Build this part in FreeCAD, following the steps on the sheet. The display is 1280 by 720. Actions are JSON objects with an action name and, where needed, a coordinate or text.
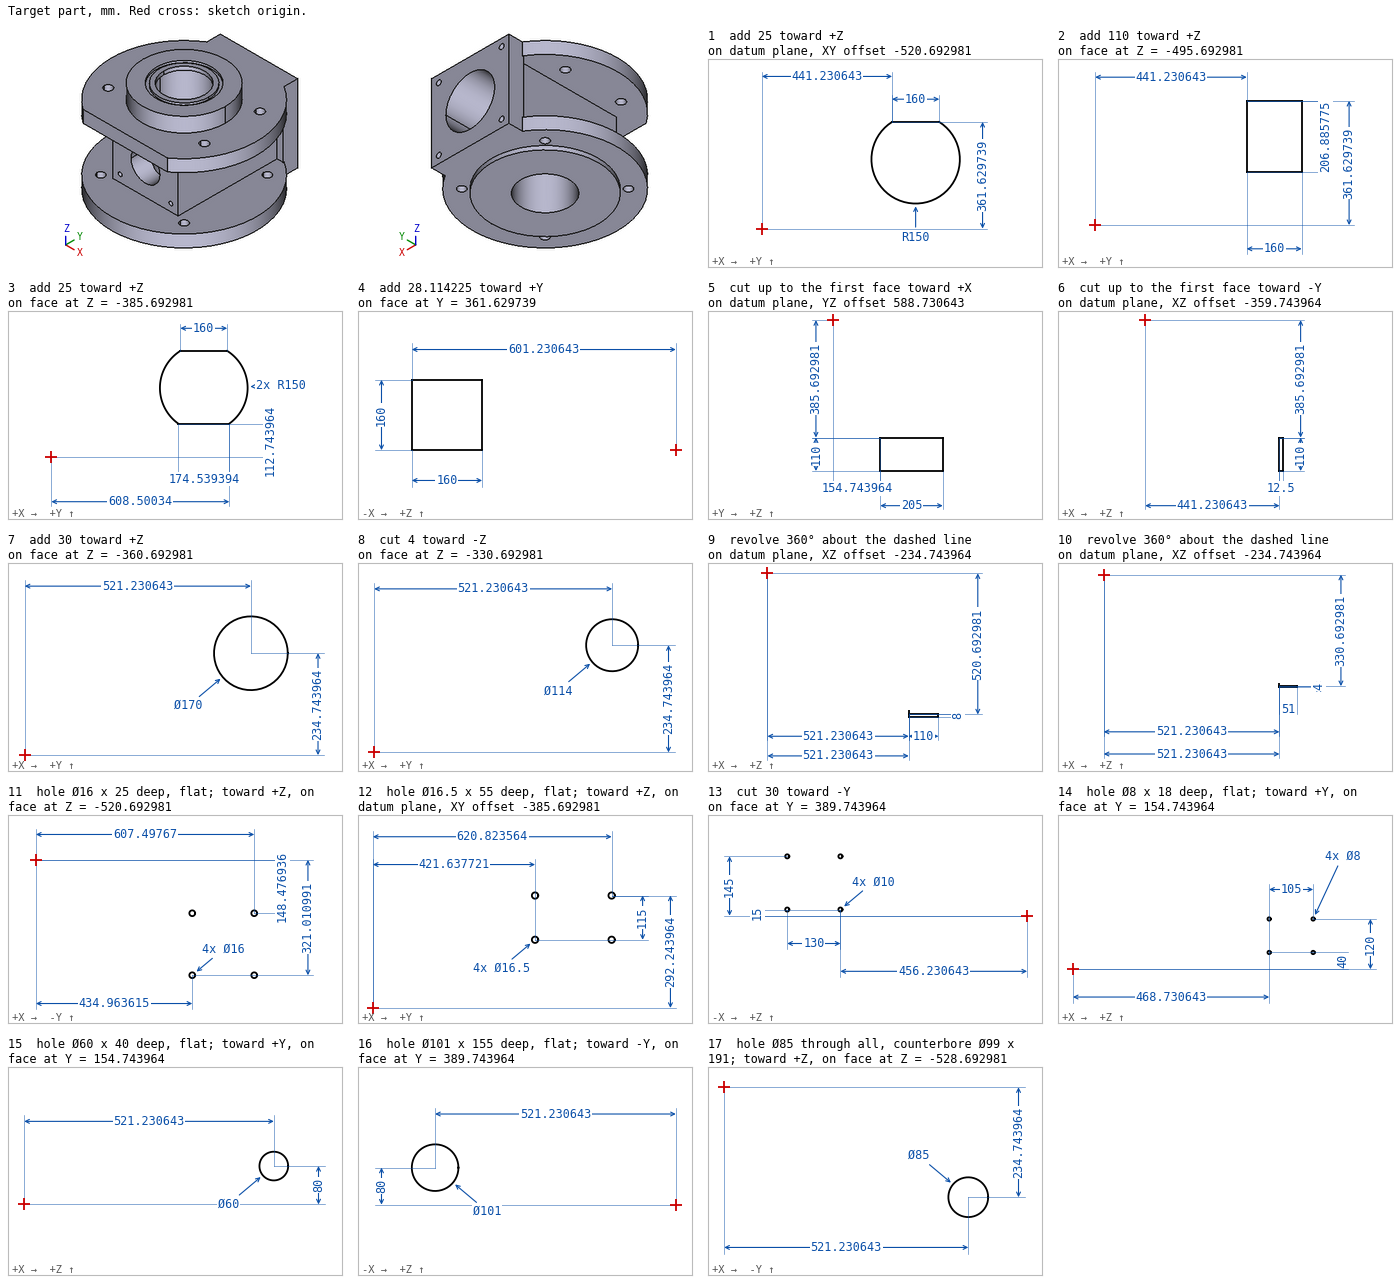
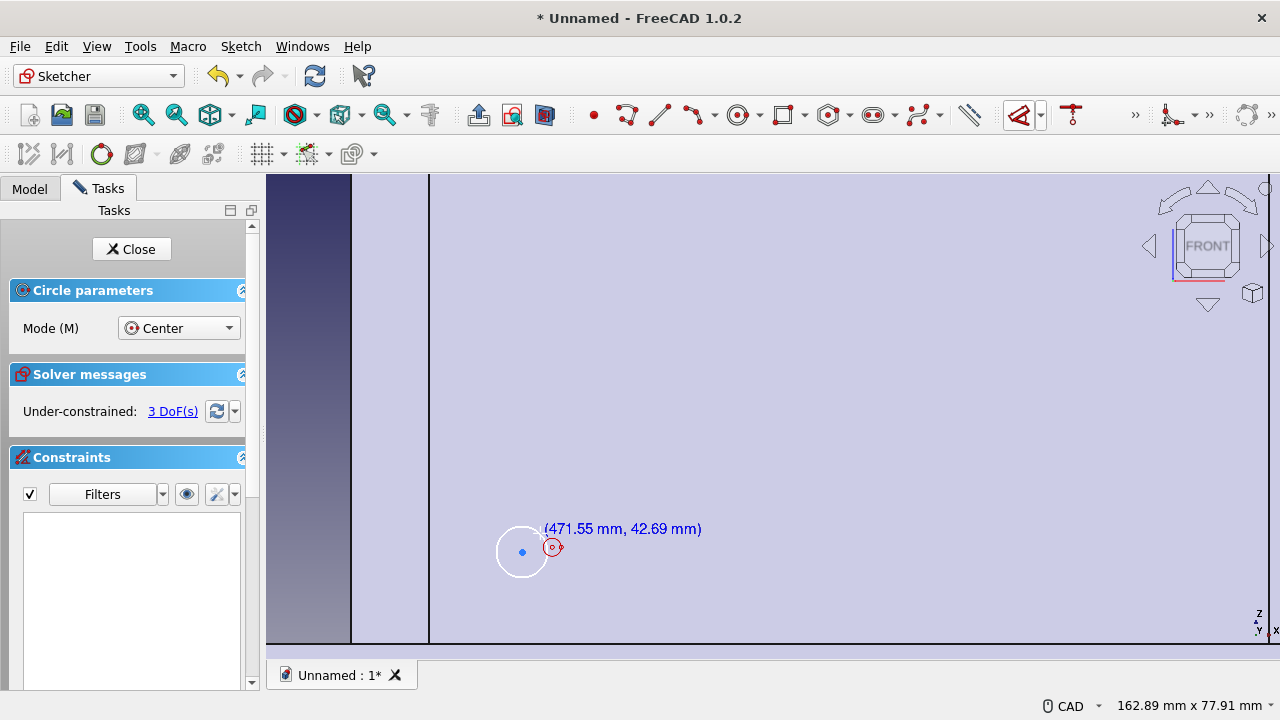
{"action": "scroll", "coordinate": [528, 556], "scroll_direction": "down", "scroll_amount": 3}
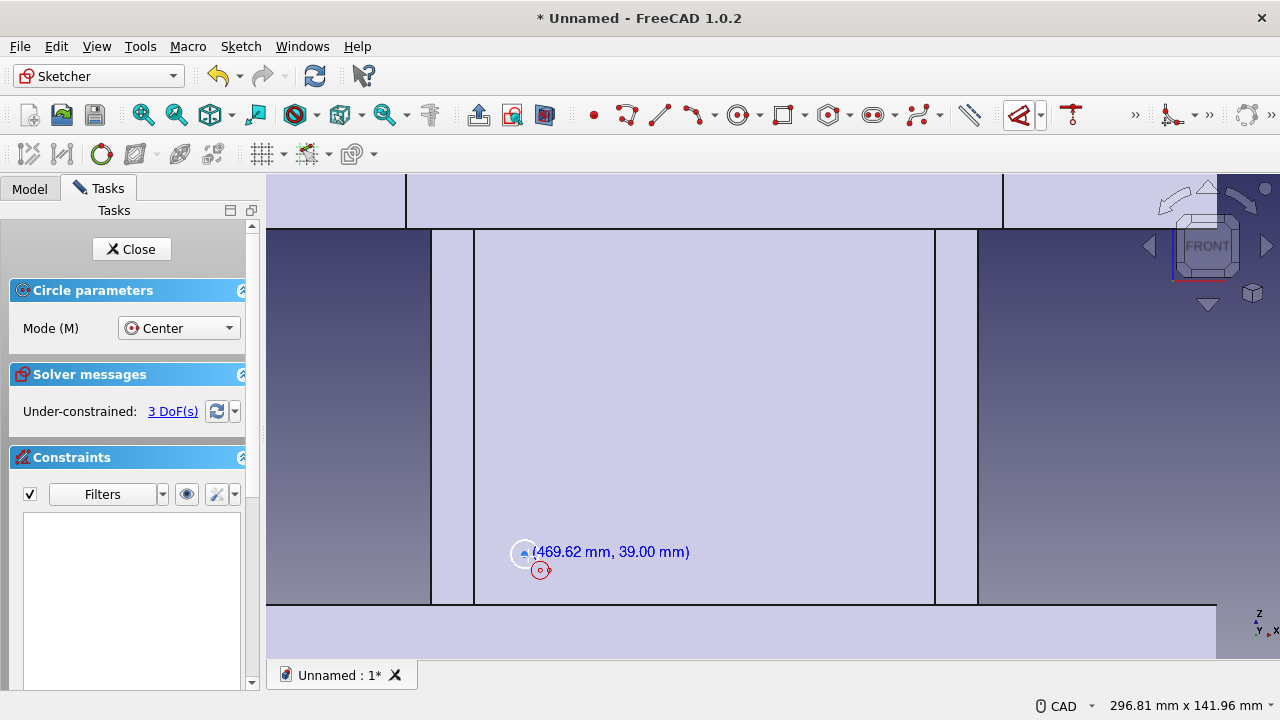
{"action": "scroll", "coordinate": [884, 280], "scroll_direction": "up", "scroll_amount": 3}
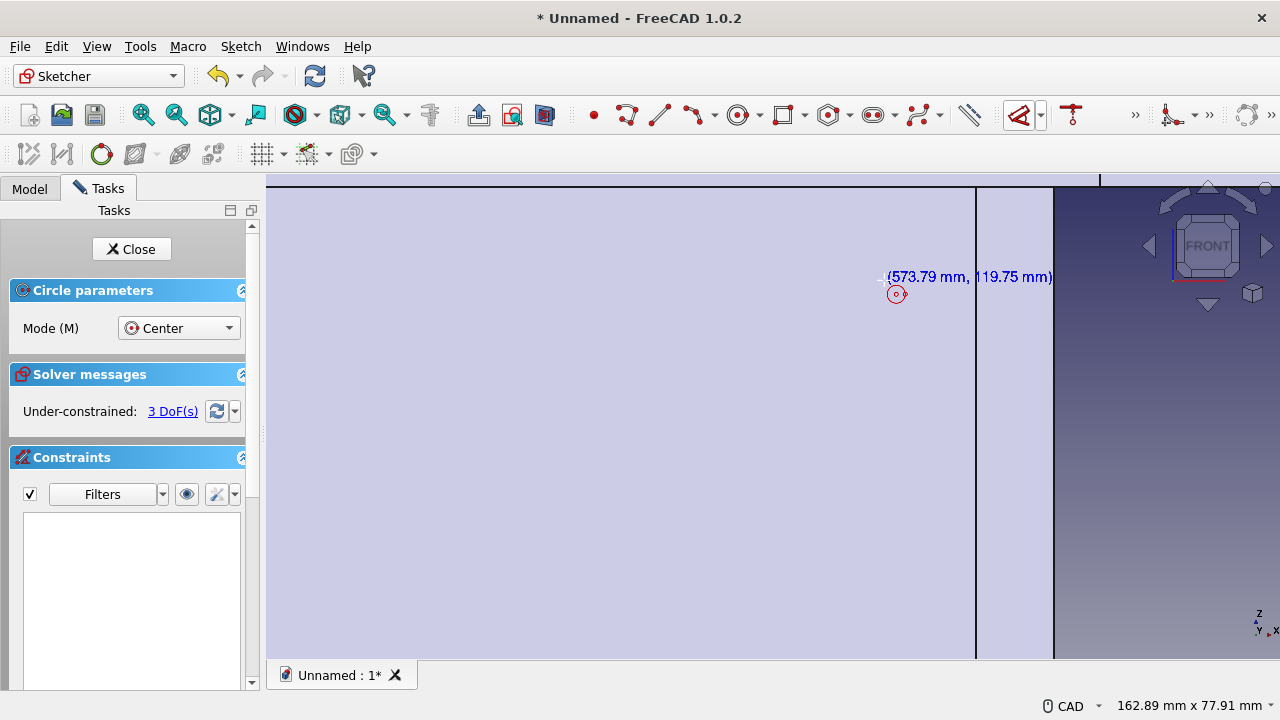
{"action": "left_click", "coordinate": [883, 280]}
{"action": "left_click", "coordinate": [901, 263]}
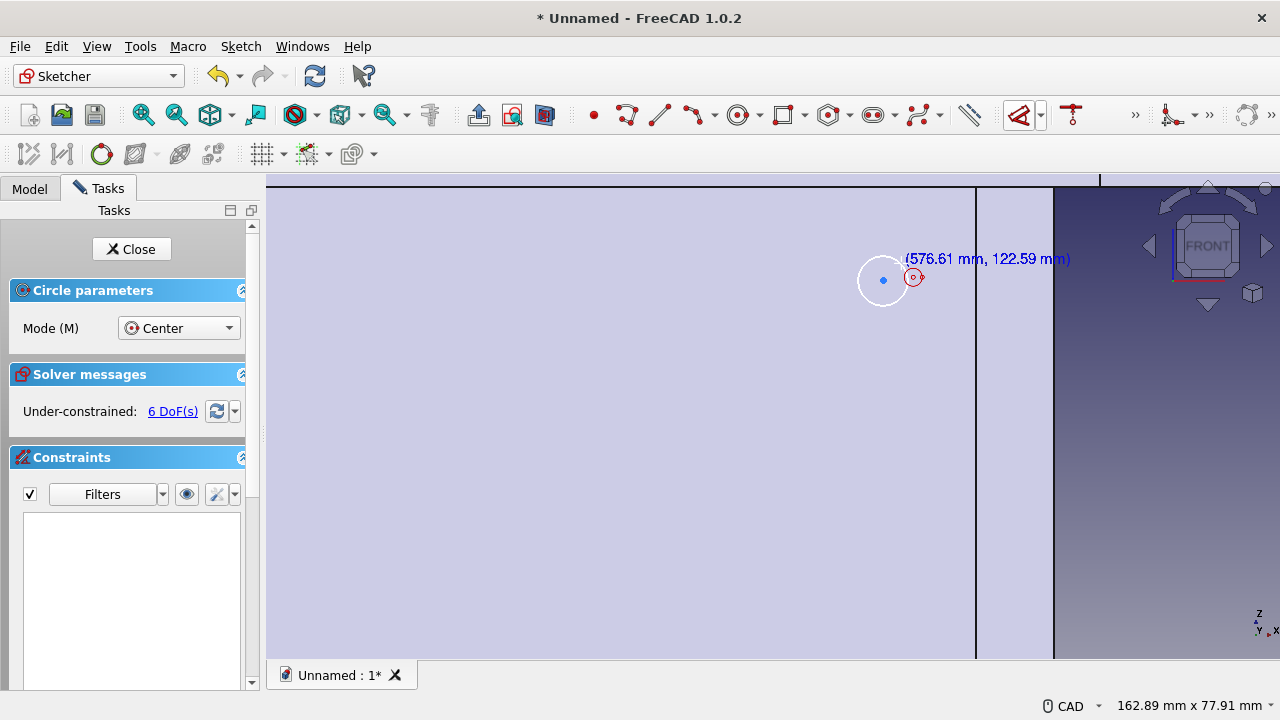
{"action": "scroll", "coordinate": [885, 280], "scroll_direction": "down", "scroll_amount": 3}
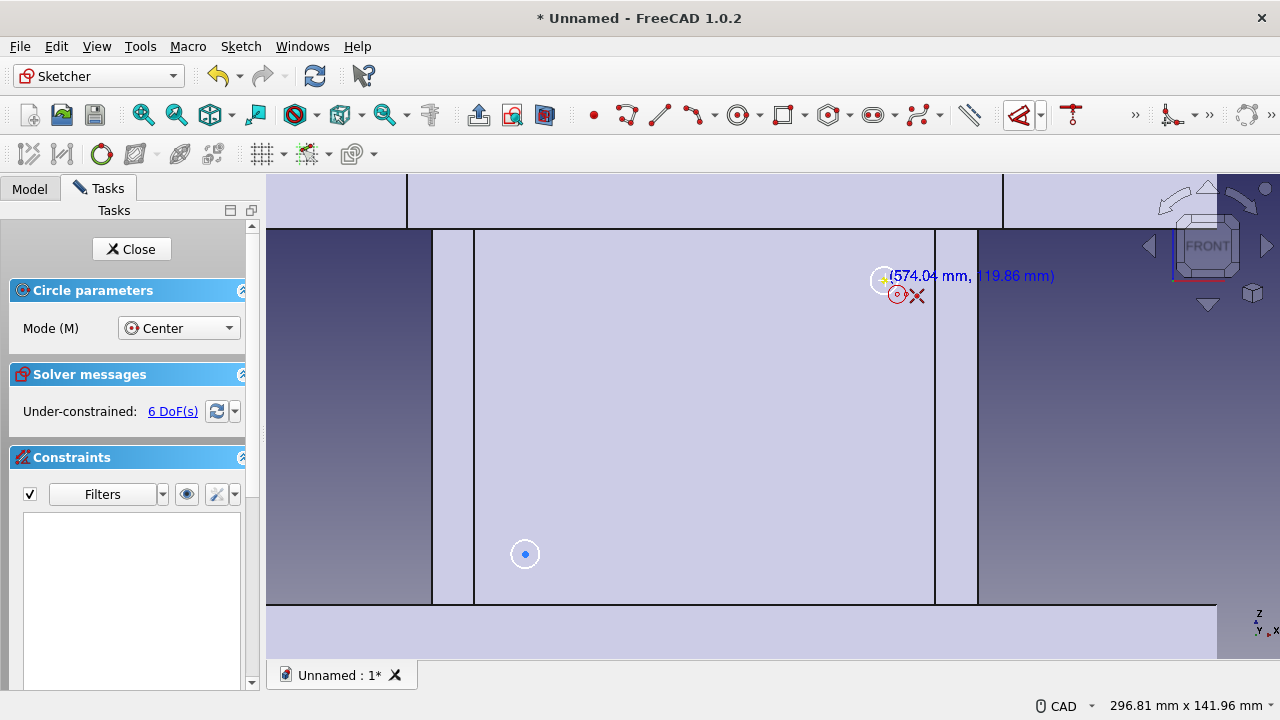
{"action": "scroll", "coordinate": [884, 553], "scroll_direction": "up", "scroll_amount": 3}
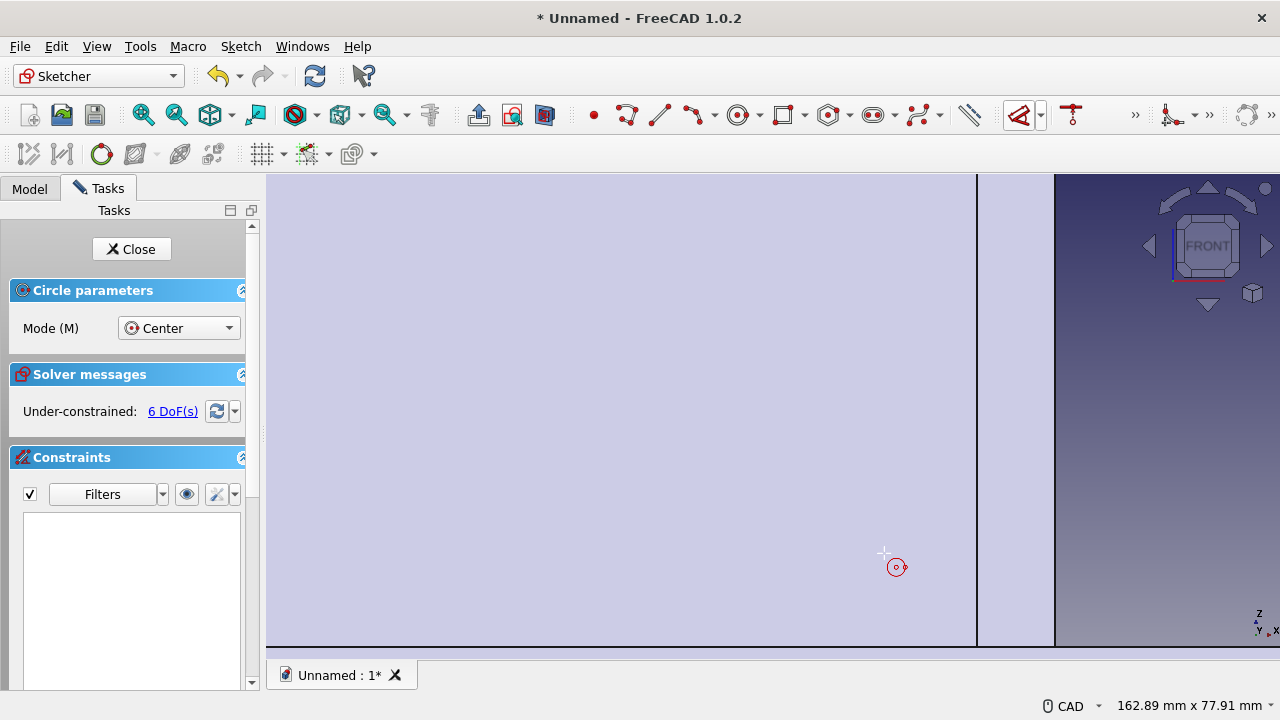
{"action": "left_click", "coordinate": [884, 553]}
{"action": "left_click", "coordinate": [902, 536]}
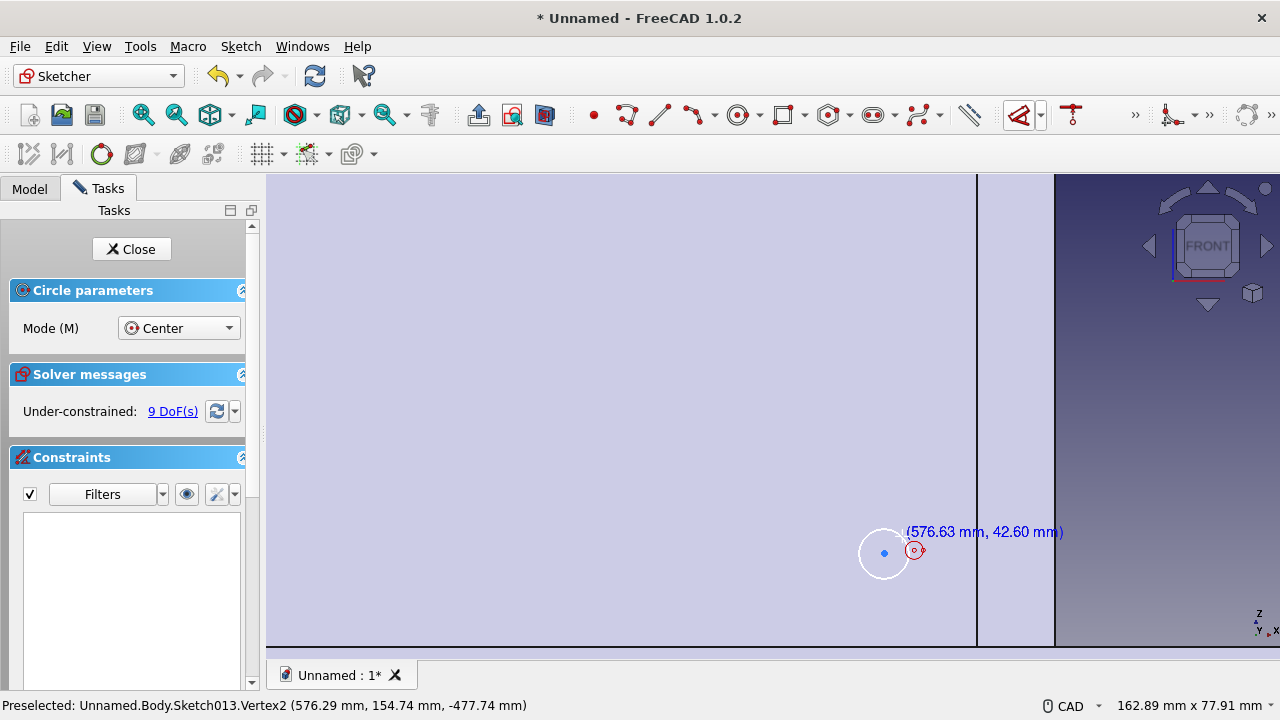
{"action": "scroll", "coordinate": [884, 553], "scroll_direction": "down", "scroll_amount": 3}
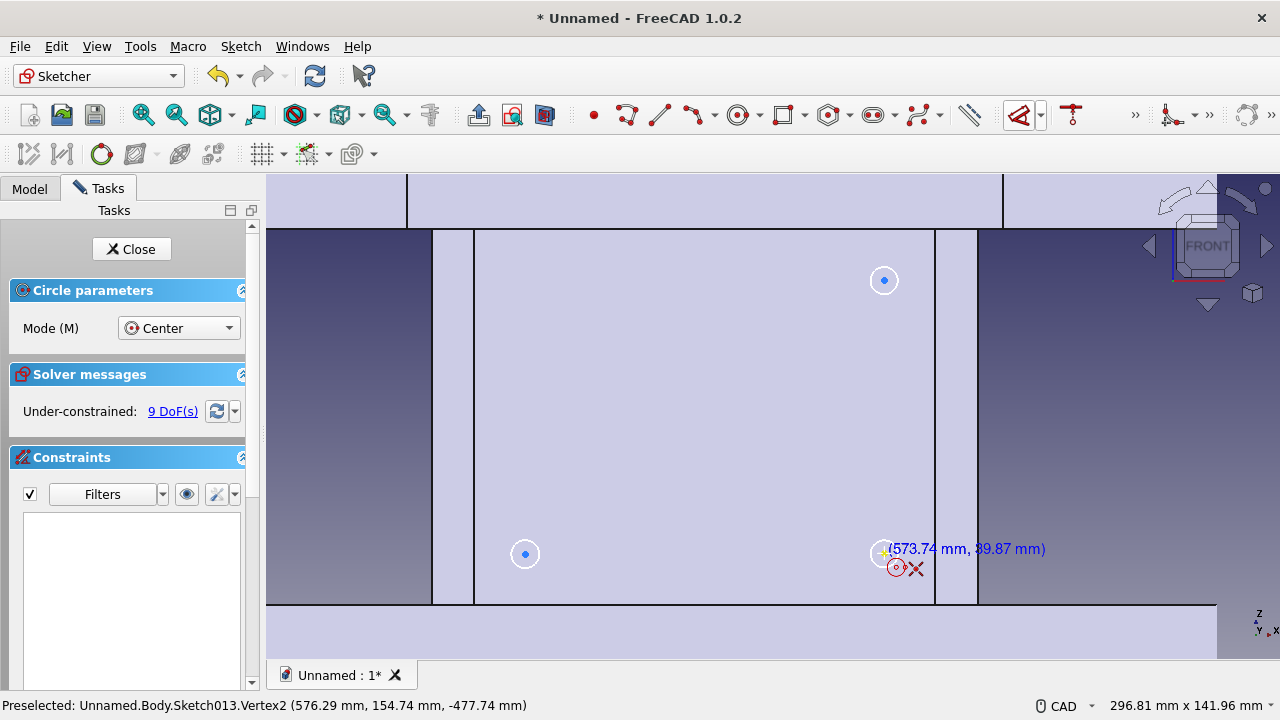
{"action": "scroll", "coordinate": [526, 280], "scroll_direction": "up", "scroll_amount": 3}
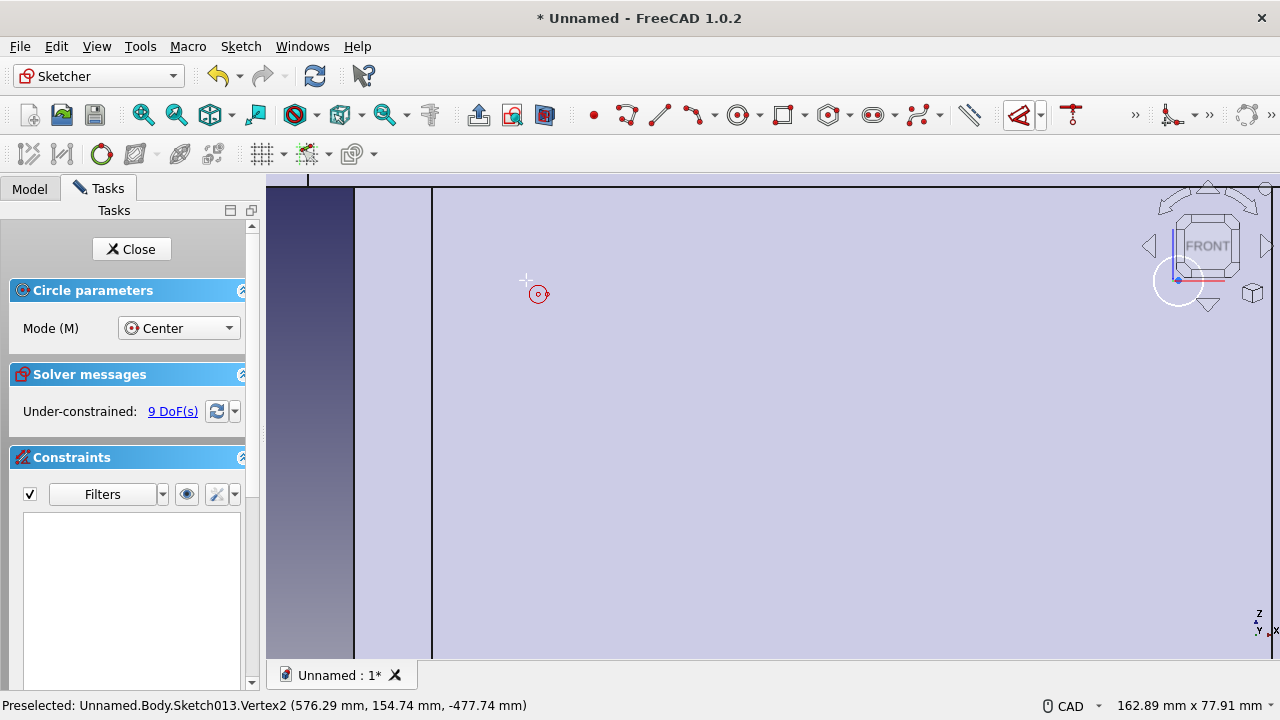
{"action": "left_click", "coordinate": [525, 280]}
{"action": "left_click", "coordinate": [543, 263]}
{"action": "key", "text": "Escape"}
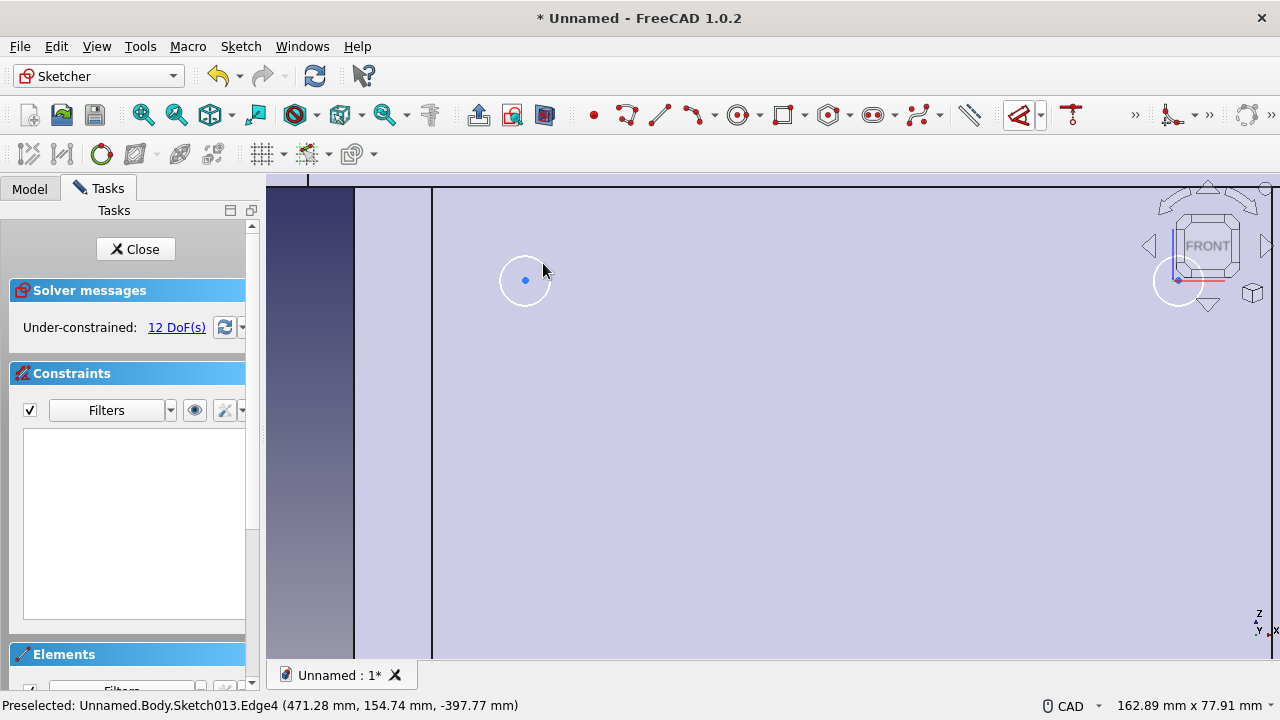
{"action": "scroll", "coordinate": [525, 280], "scroll_direction": "down", "scroll_amount": 3}